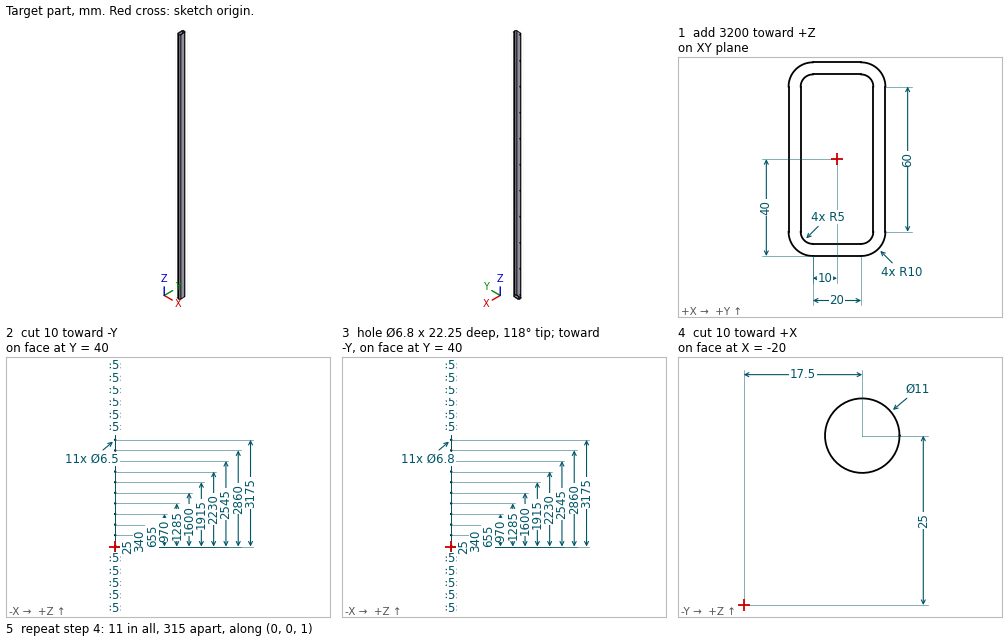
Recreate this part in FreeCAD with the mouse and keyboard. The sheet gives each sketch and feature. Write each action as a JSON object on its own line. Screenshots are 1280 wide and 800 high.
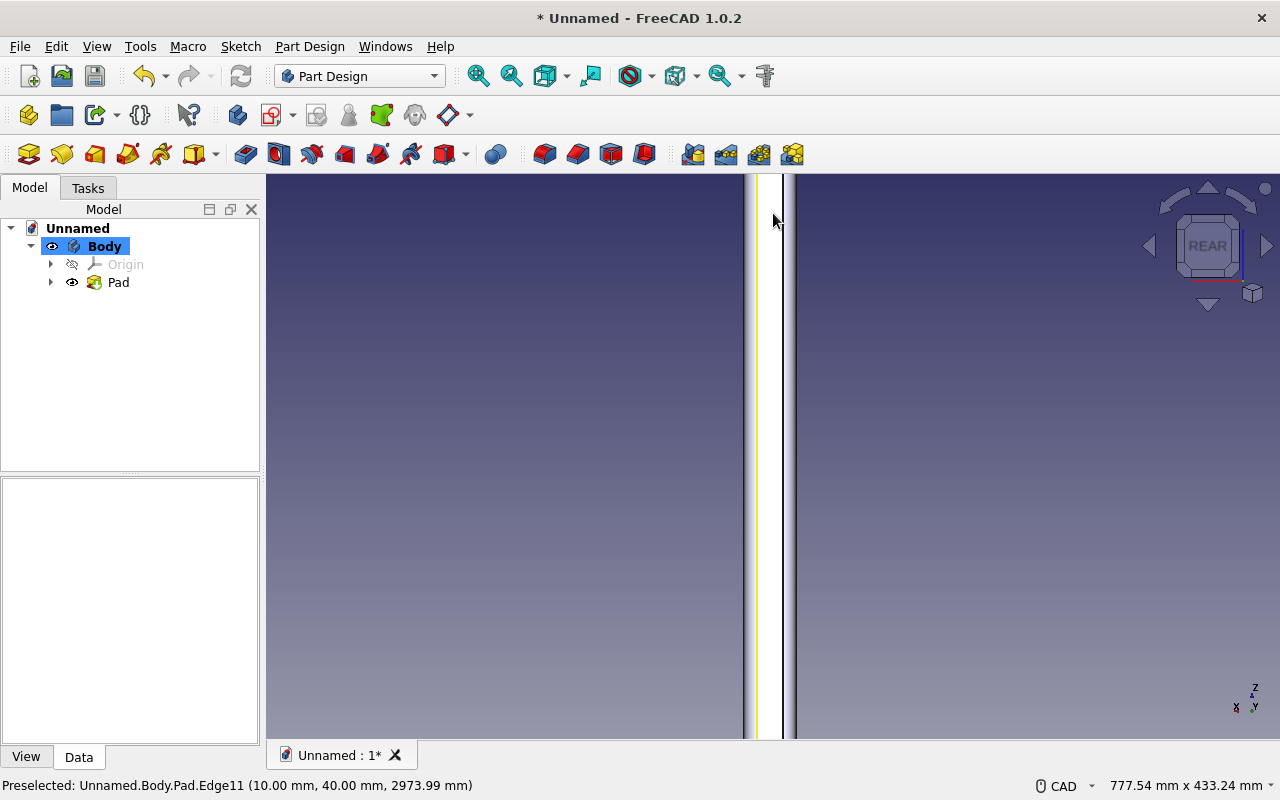
{"action": "left_click", "coordinate": [770, 222]}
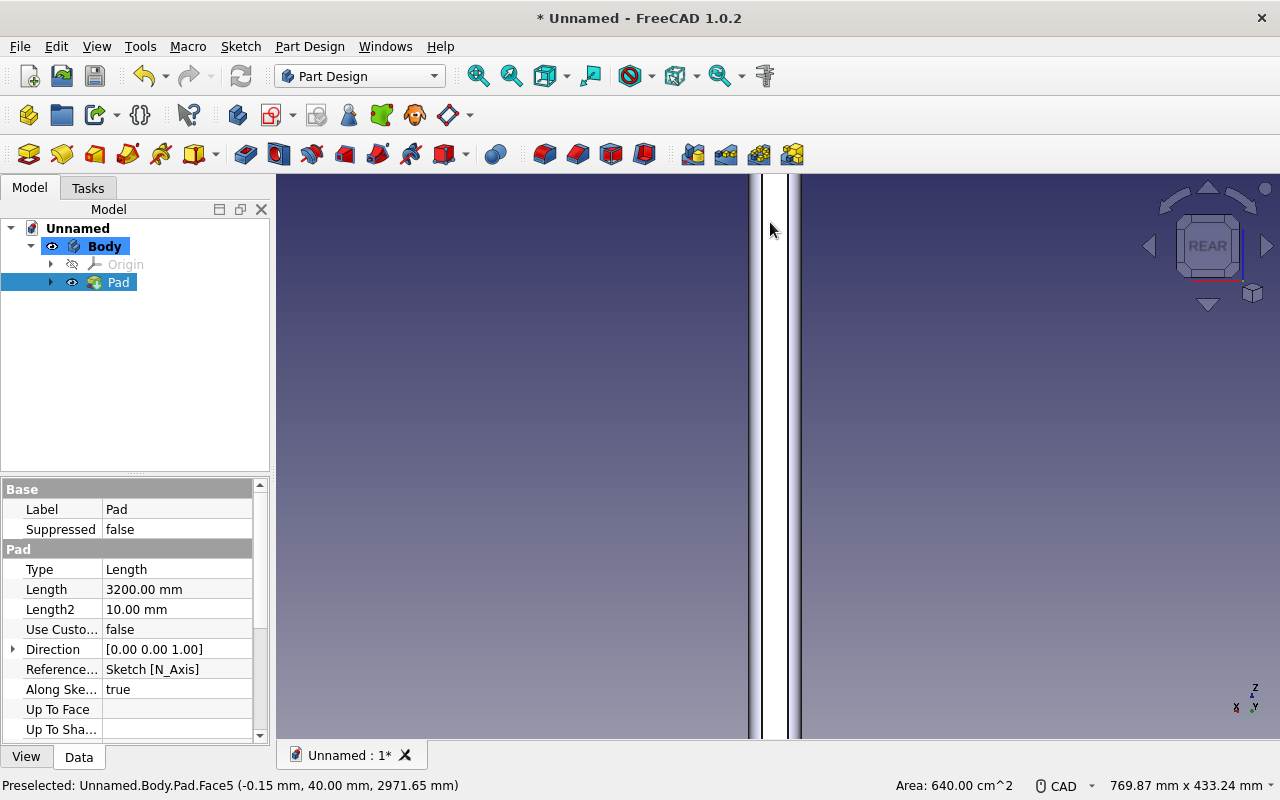
{"action": "left_click", "coordinate": [270, 116]}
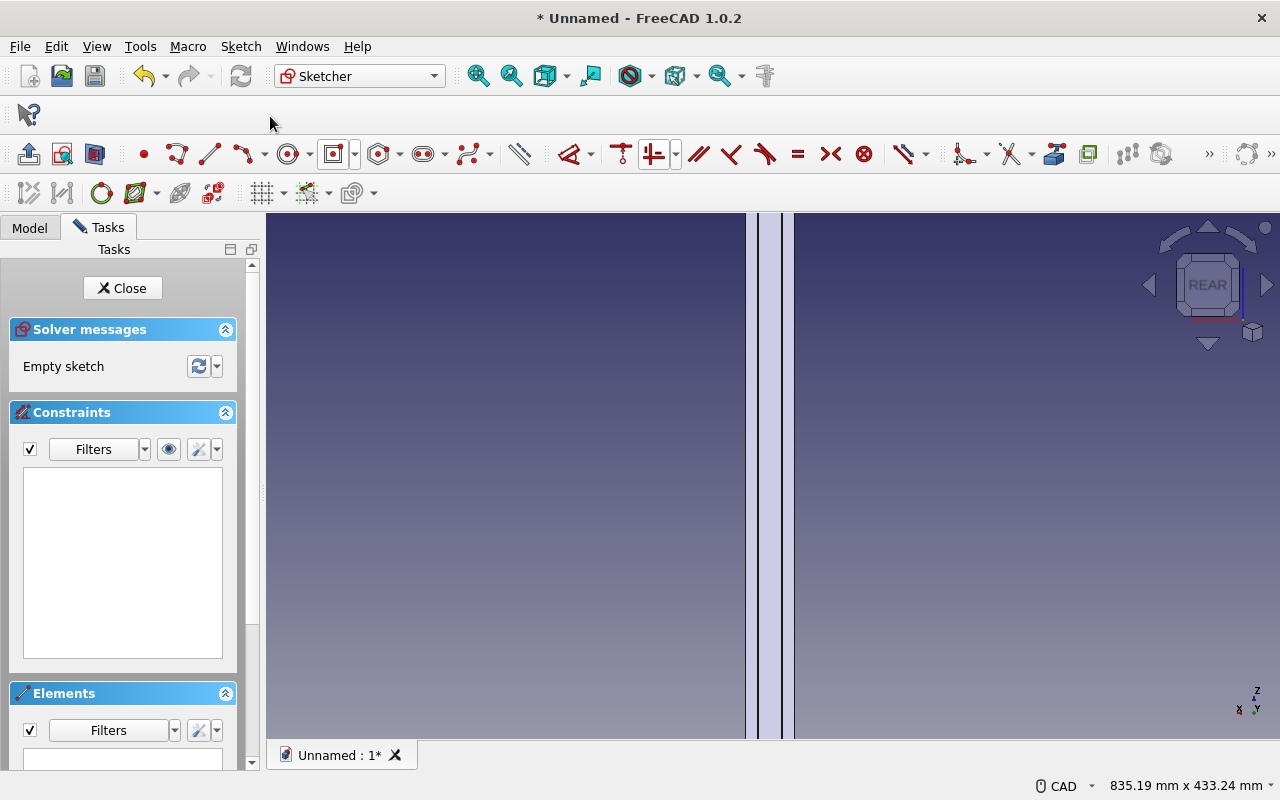
{"action": "scroll", "coordinate": [697, 330], "scroll_direction": "down", "scroll_amount": 12}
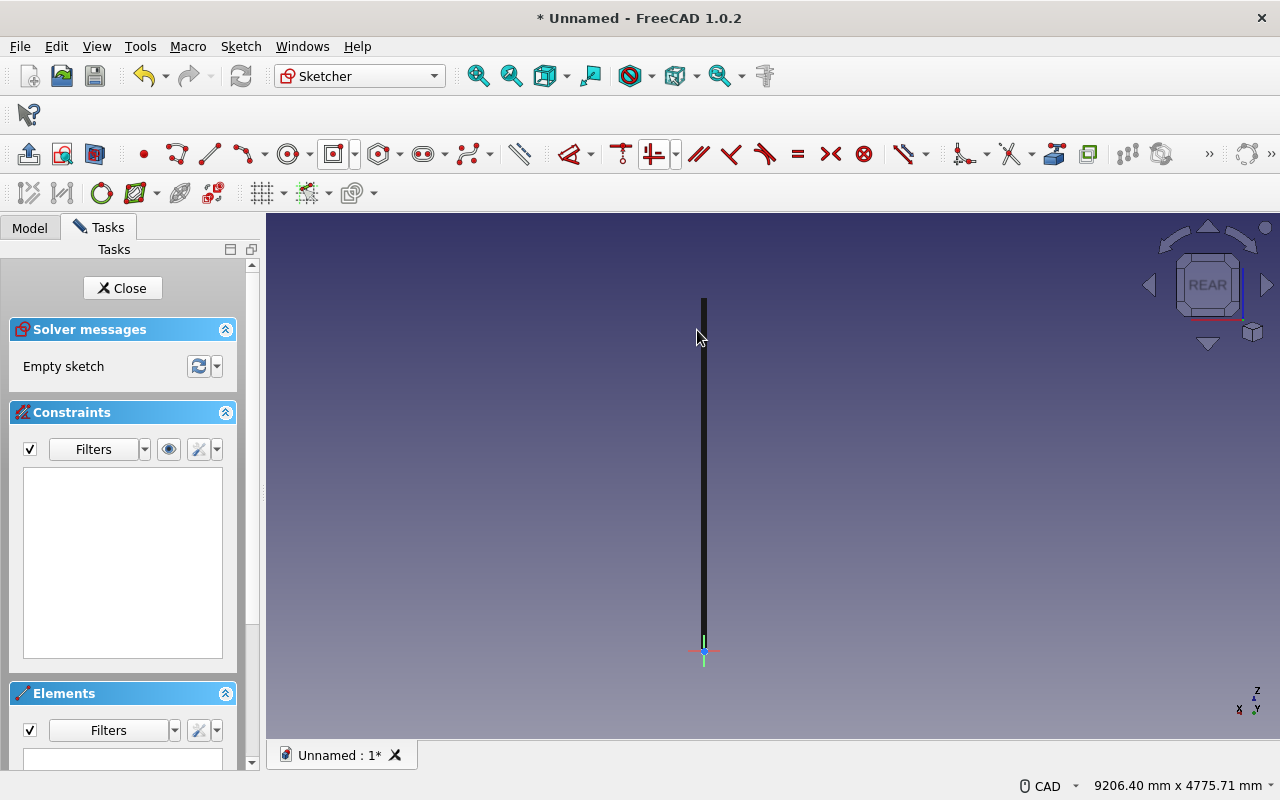
{"action": "left_click", "coordinate": [288, 154]}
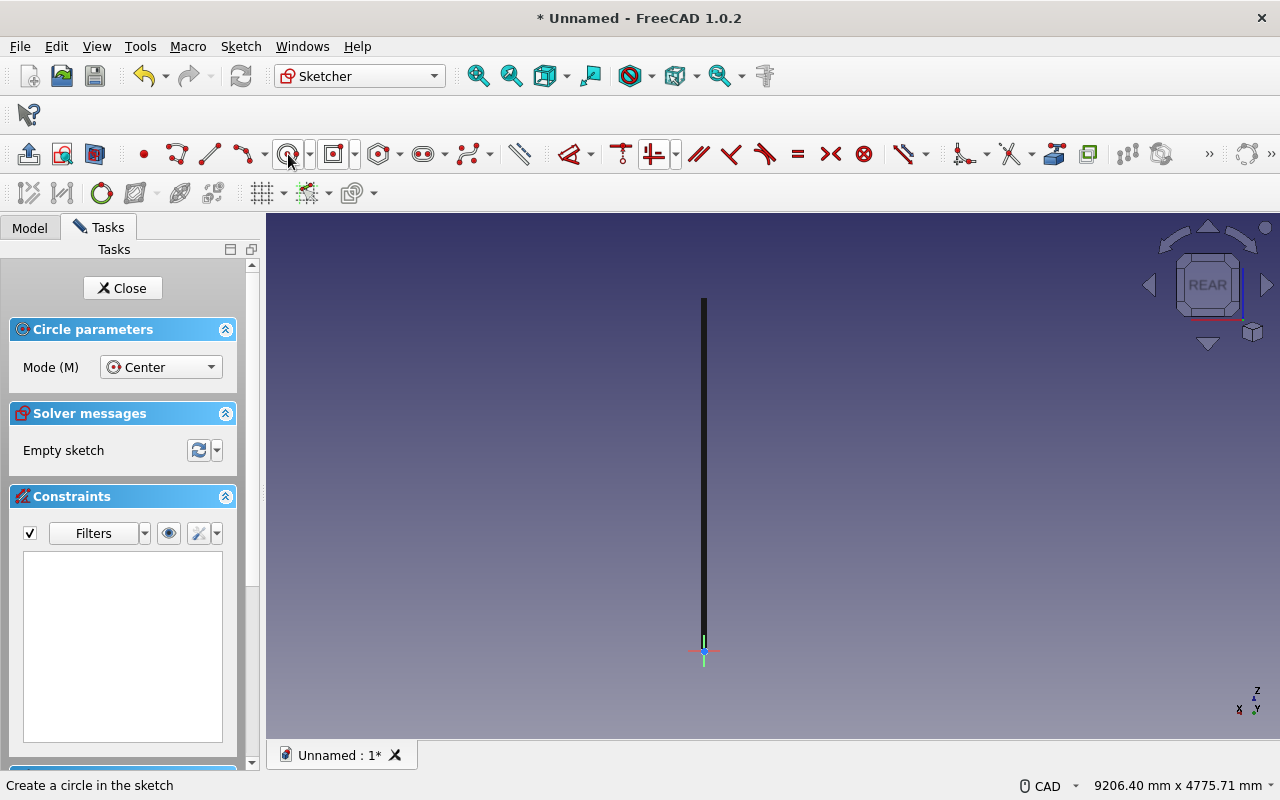
{"action": "scroll", "coordinate": [705, 301], "scroll_direction": "up", "scroll_amount": 21}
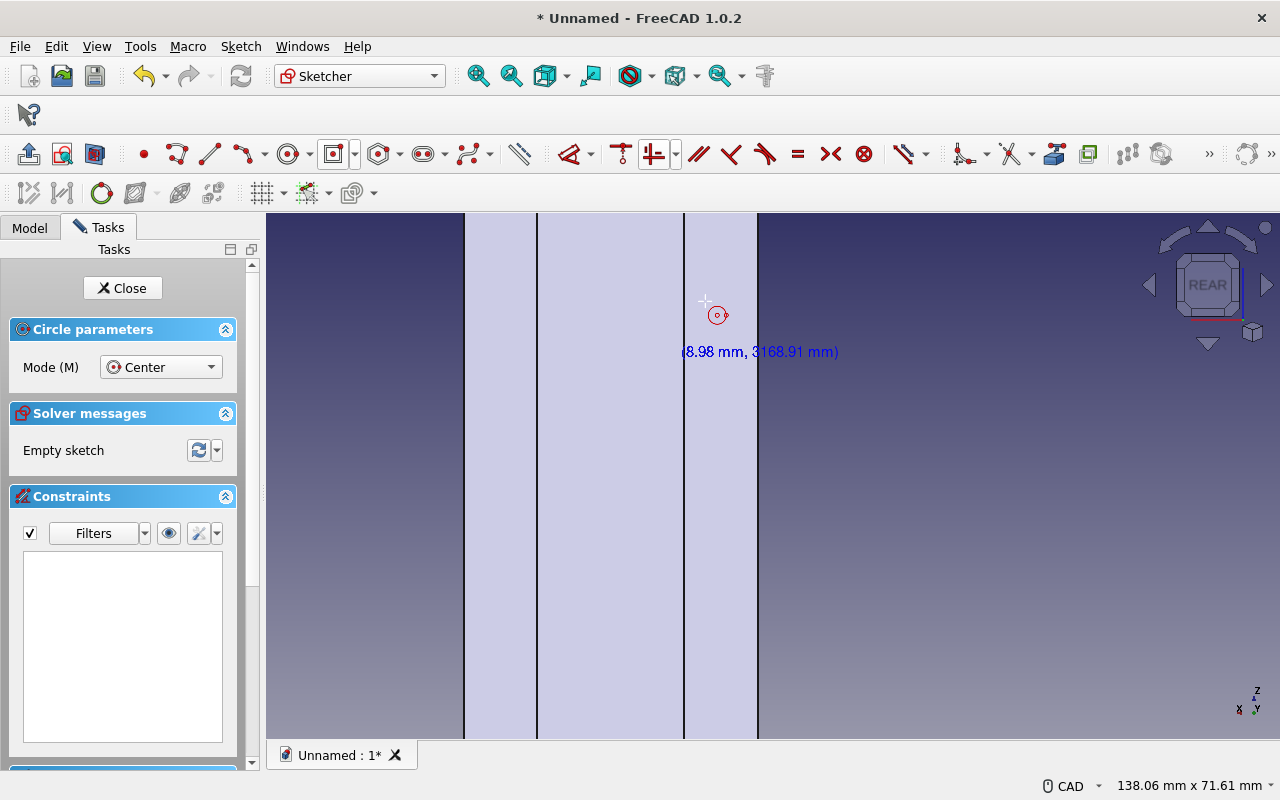
{"action": "left_click", "coordinate": [647, 312]}
{"action": "left_click", "coordinate": [664, 295]}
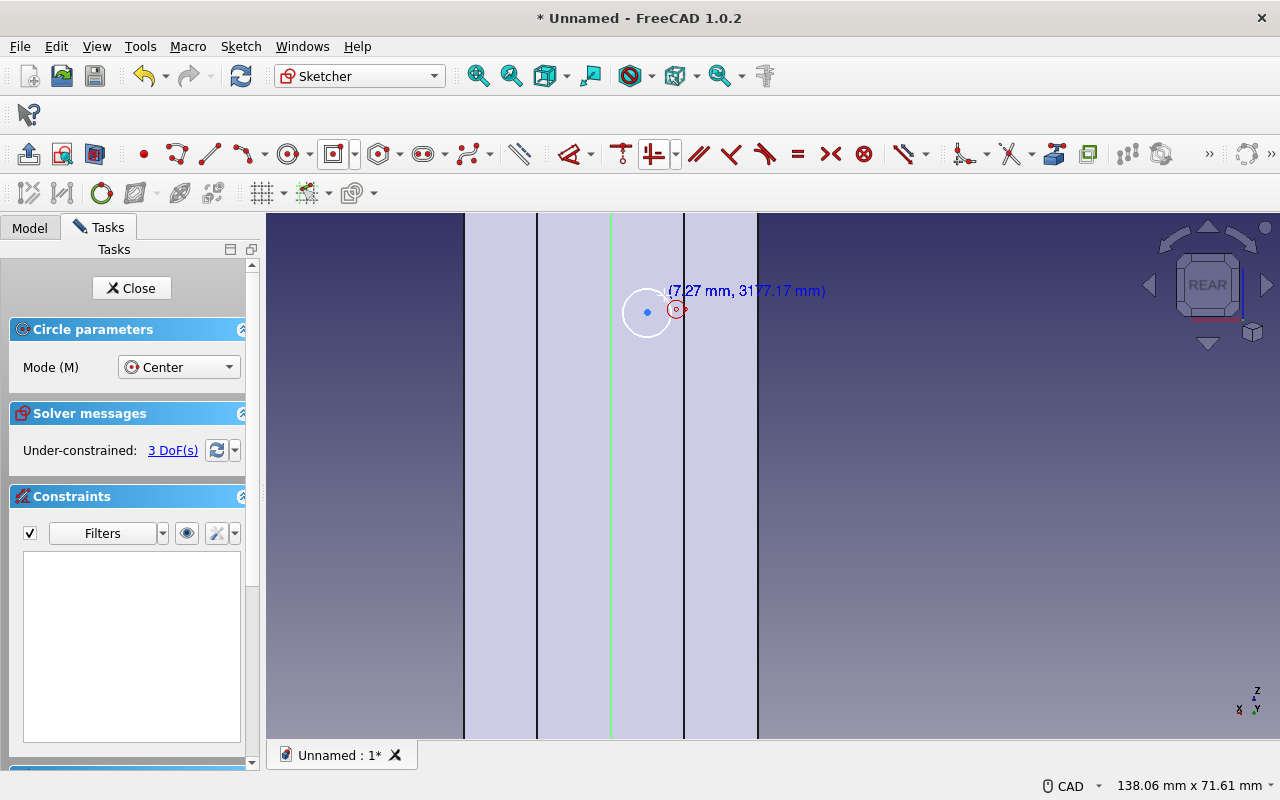
{"action": "scroll", "coordinate": [704, 476], "scroll_direction": "down", "scroll_amount": 15}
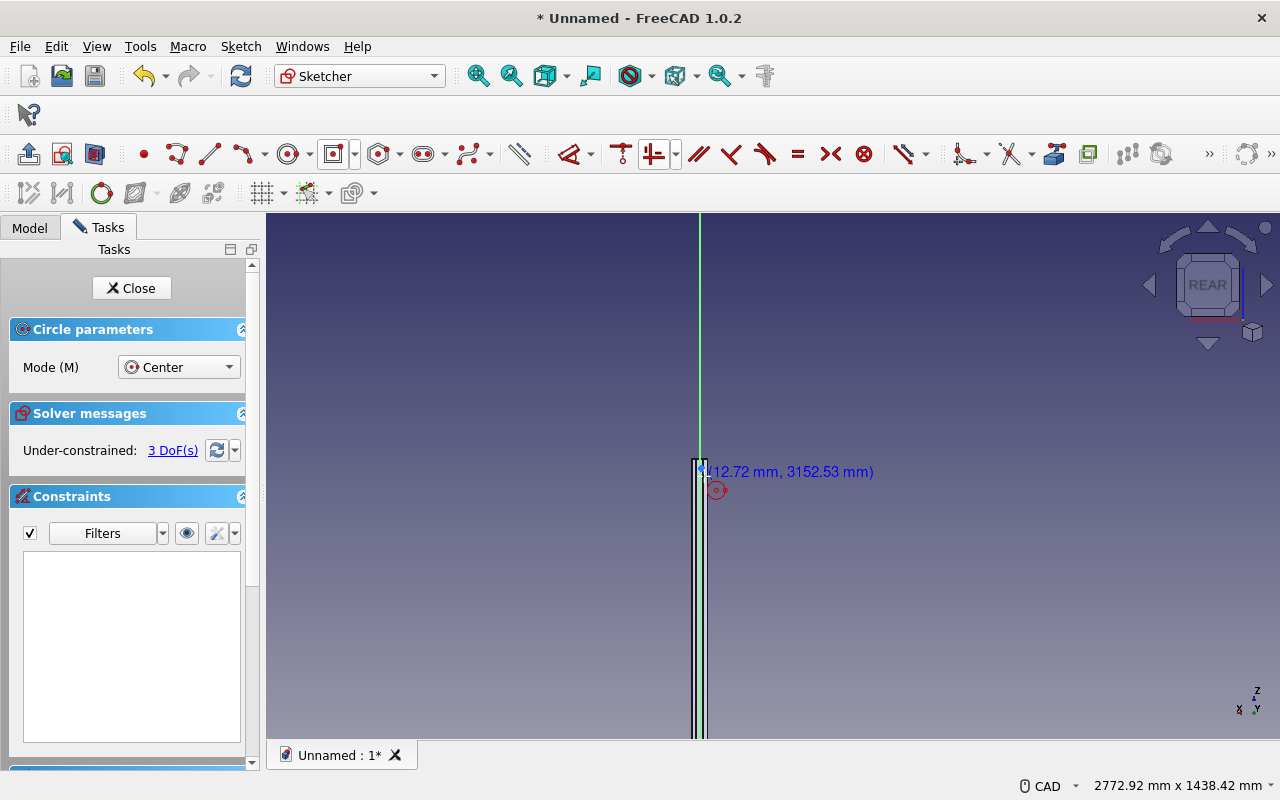
{"action": "scroll", "coordinate": [706, 241], "scroll_direction": "down", "scroll_amount": 6}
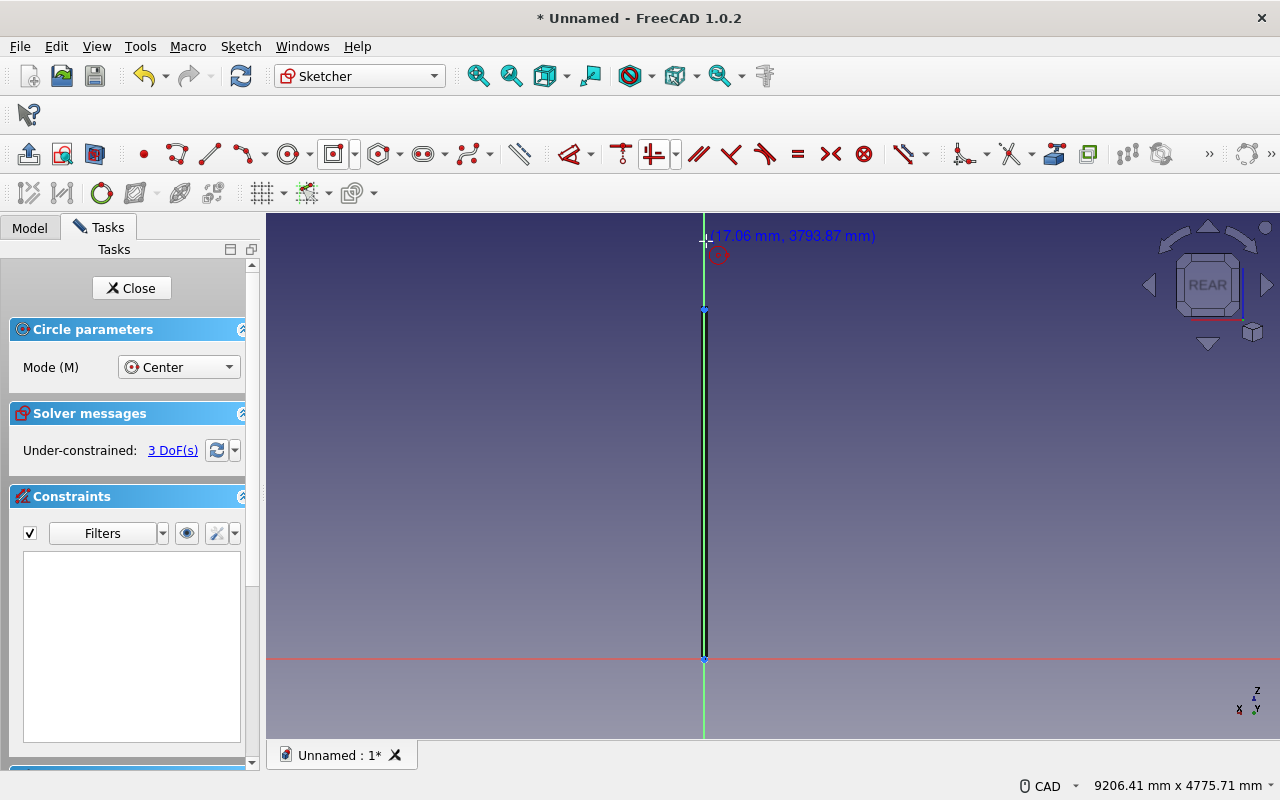
{"action": "scroll", "coordinate": [705, 344], "scroll_direction": "up", "scroll_amount": 21}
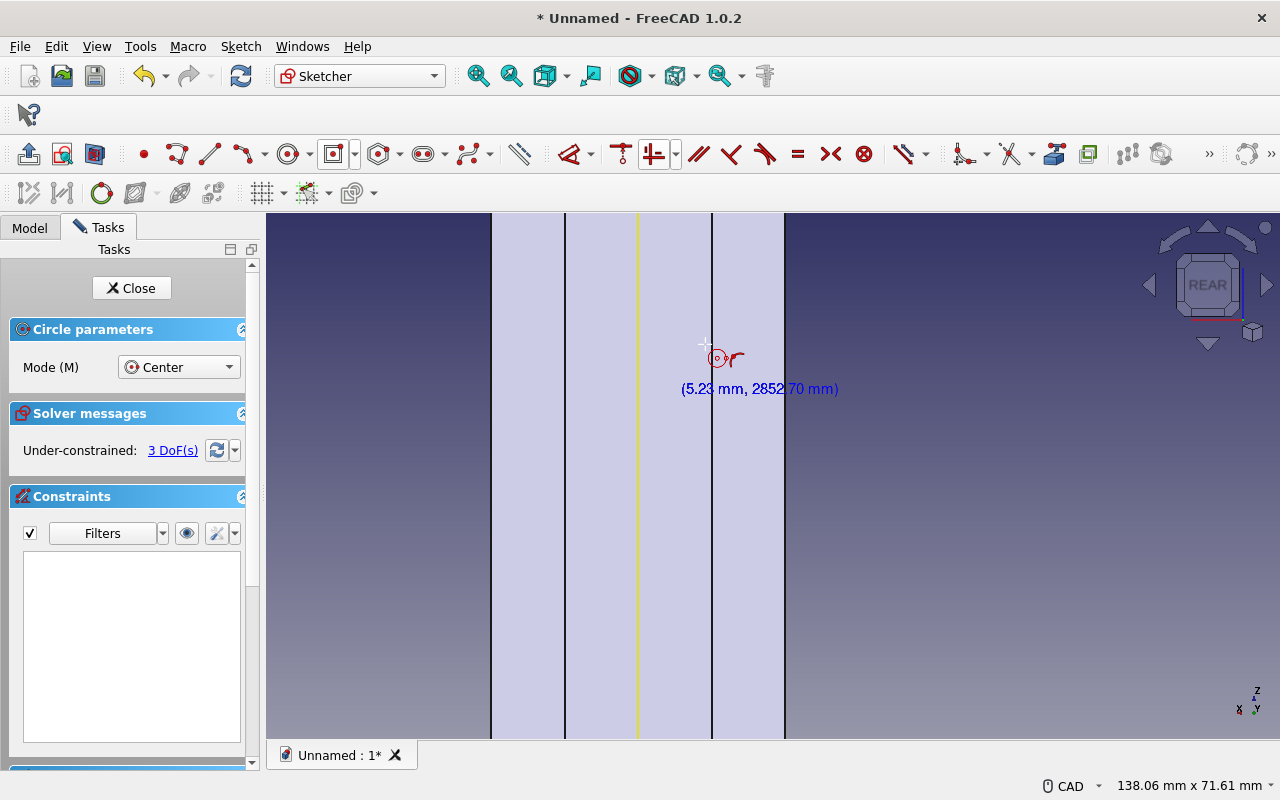
{"action": "left_click", "coordinate": [675, 341]}
{"action": "left_click", "coordinate": [692, 324]}